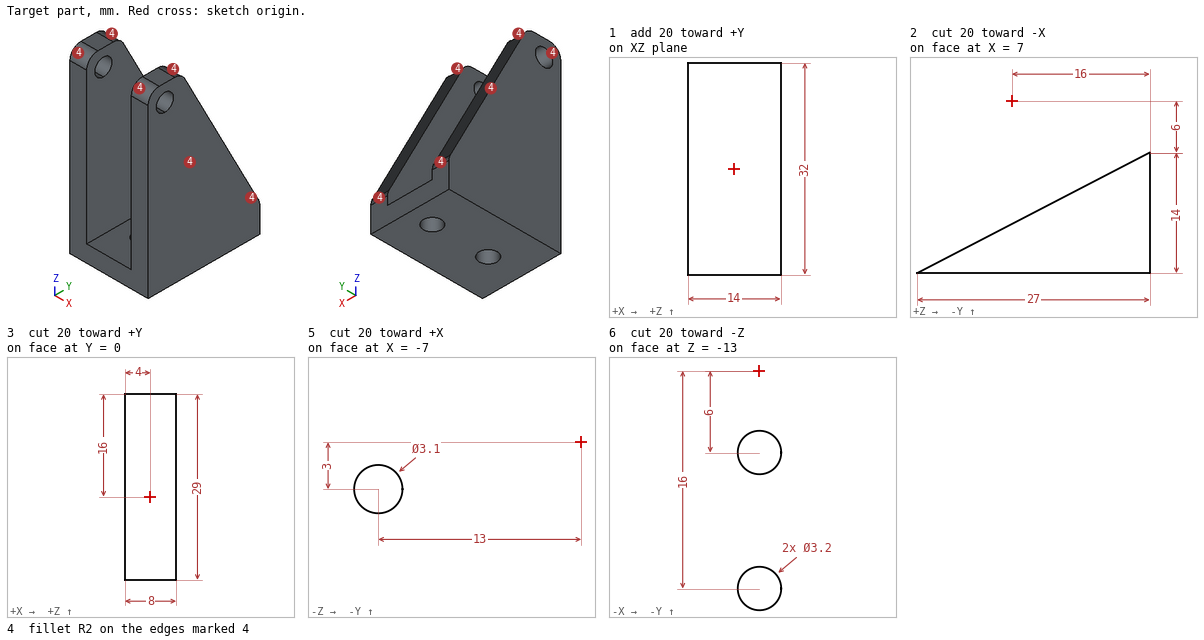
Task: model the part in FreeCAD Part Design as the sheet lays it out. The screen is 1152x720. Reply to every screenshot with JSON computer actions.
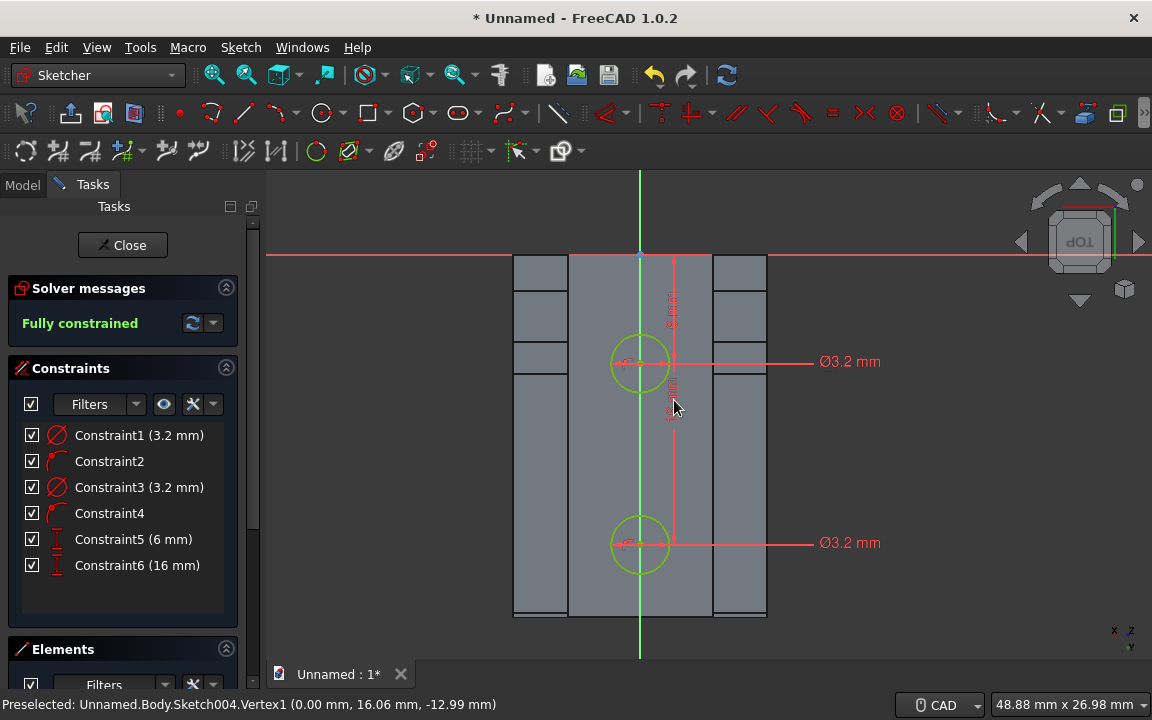
{"action": "left_click", "coordinate": [123, 245]}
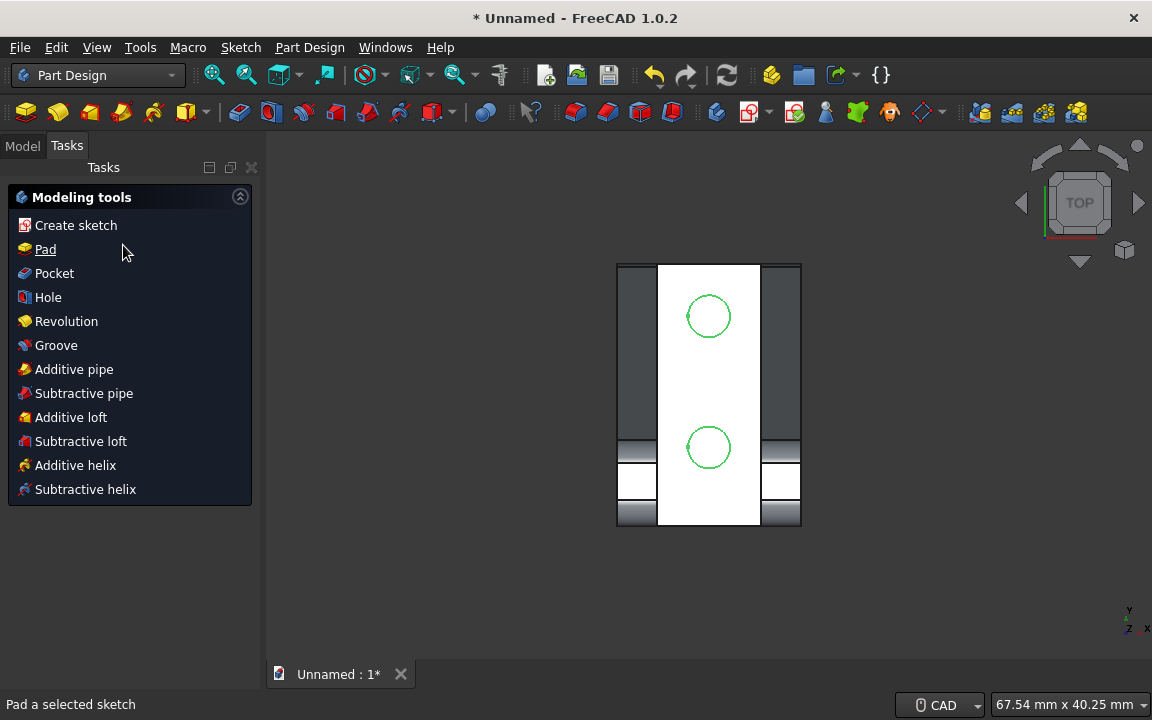
{"action": "left_click", "coordinate": [240, 112]}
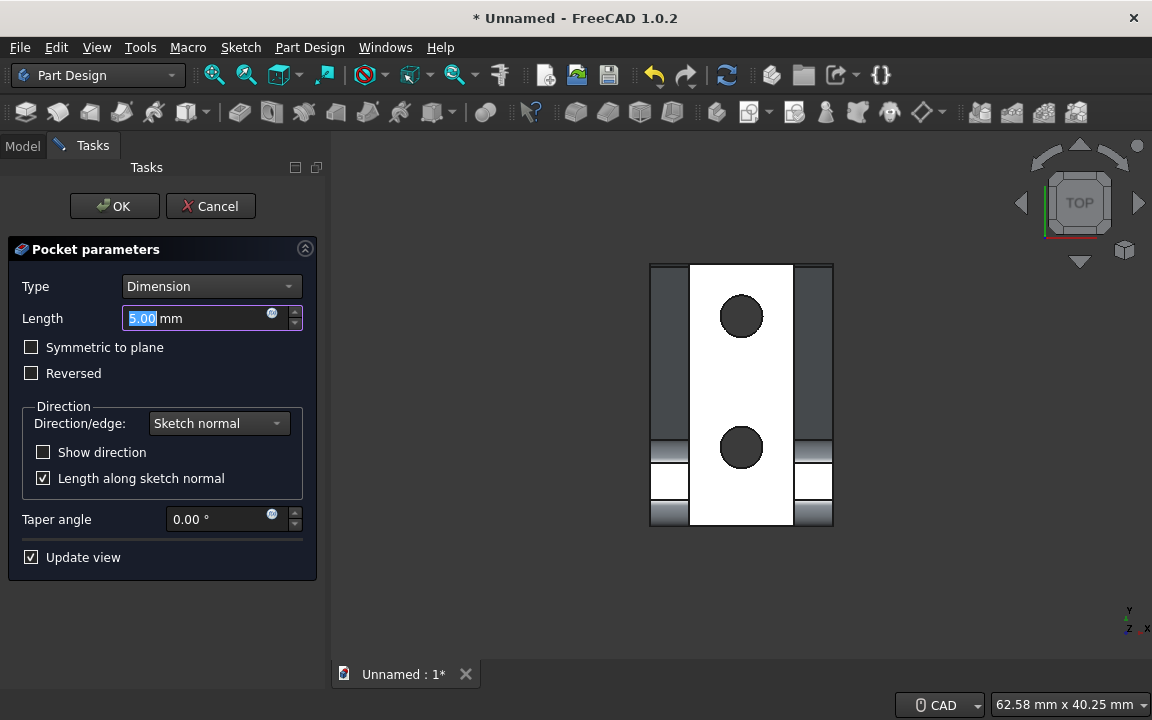
{"action": "type", "text": "20"}
{"action": "key", "text": "Tab"}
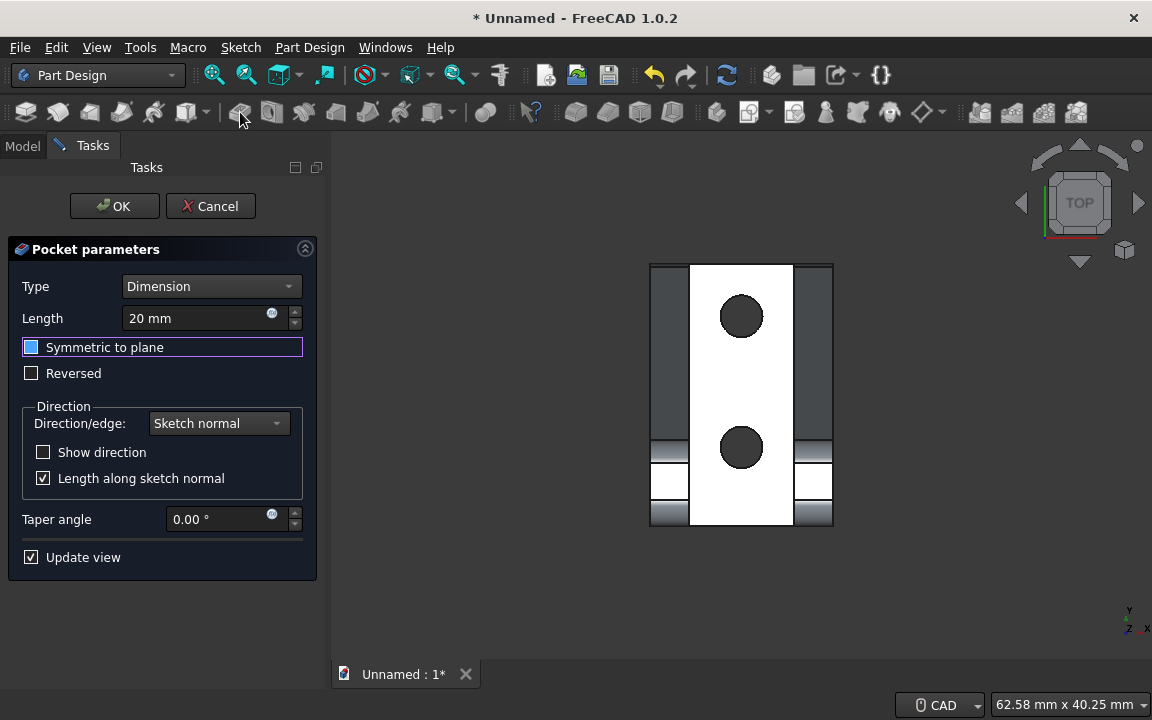
{"action": "left_click", "coordinate": [115, 206]}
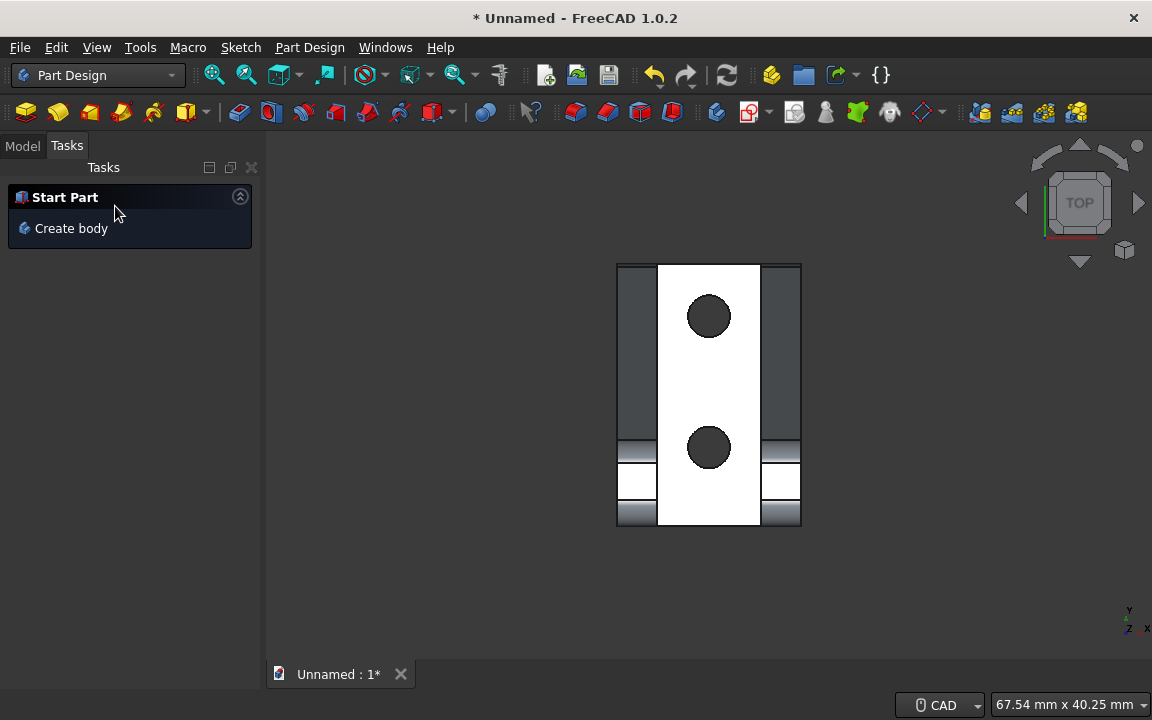
{"action": "key", "text": "0"}